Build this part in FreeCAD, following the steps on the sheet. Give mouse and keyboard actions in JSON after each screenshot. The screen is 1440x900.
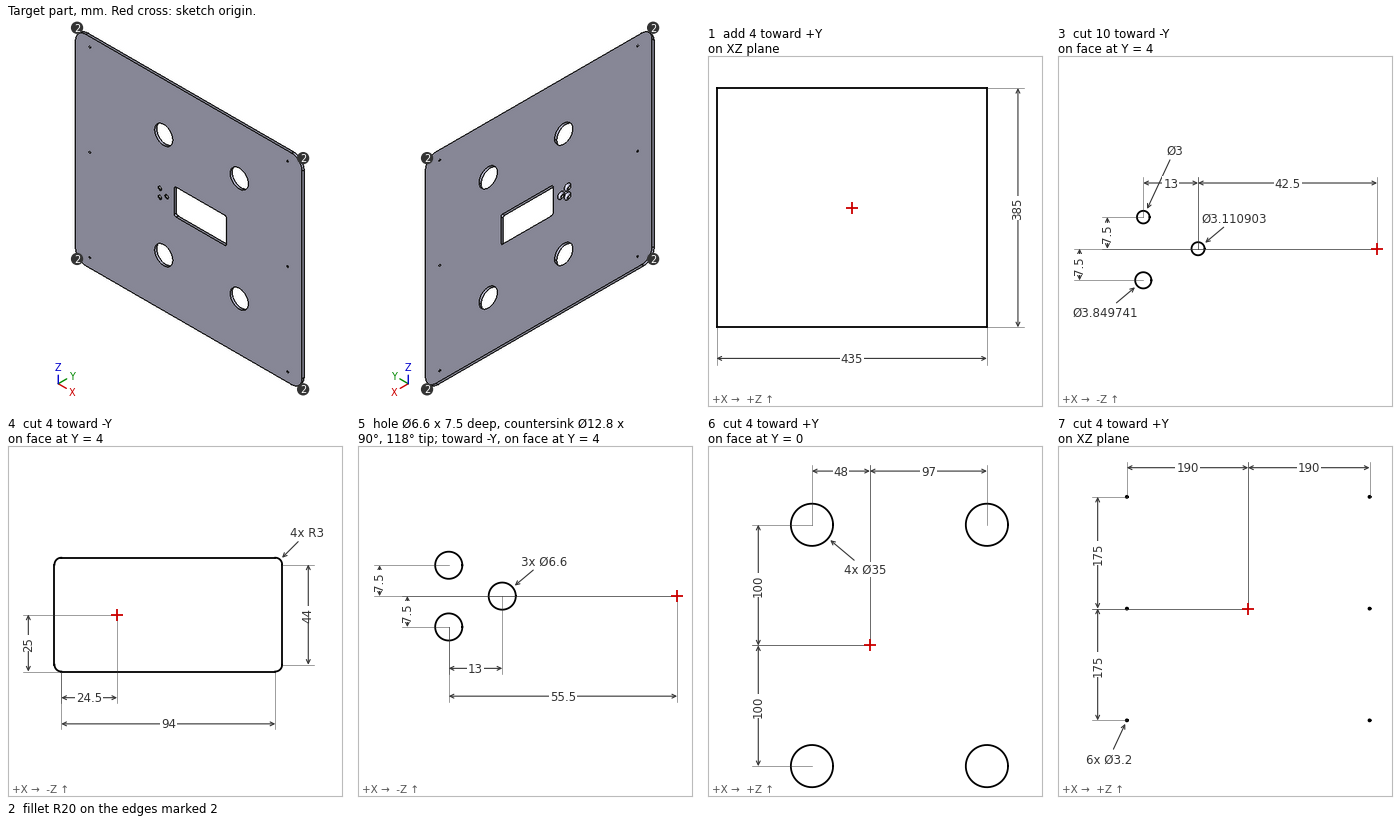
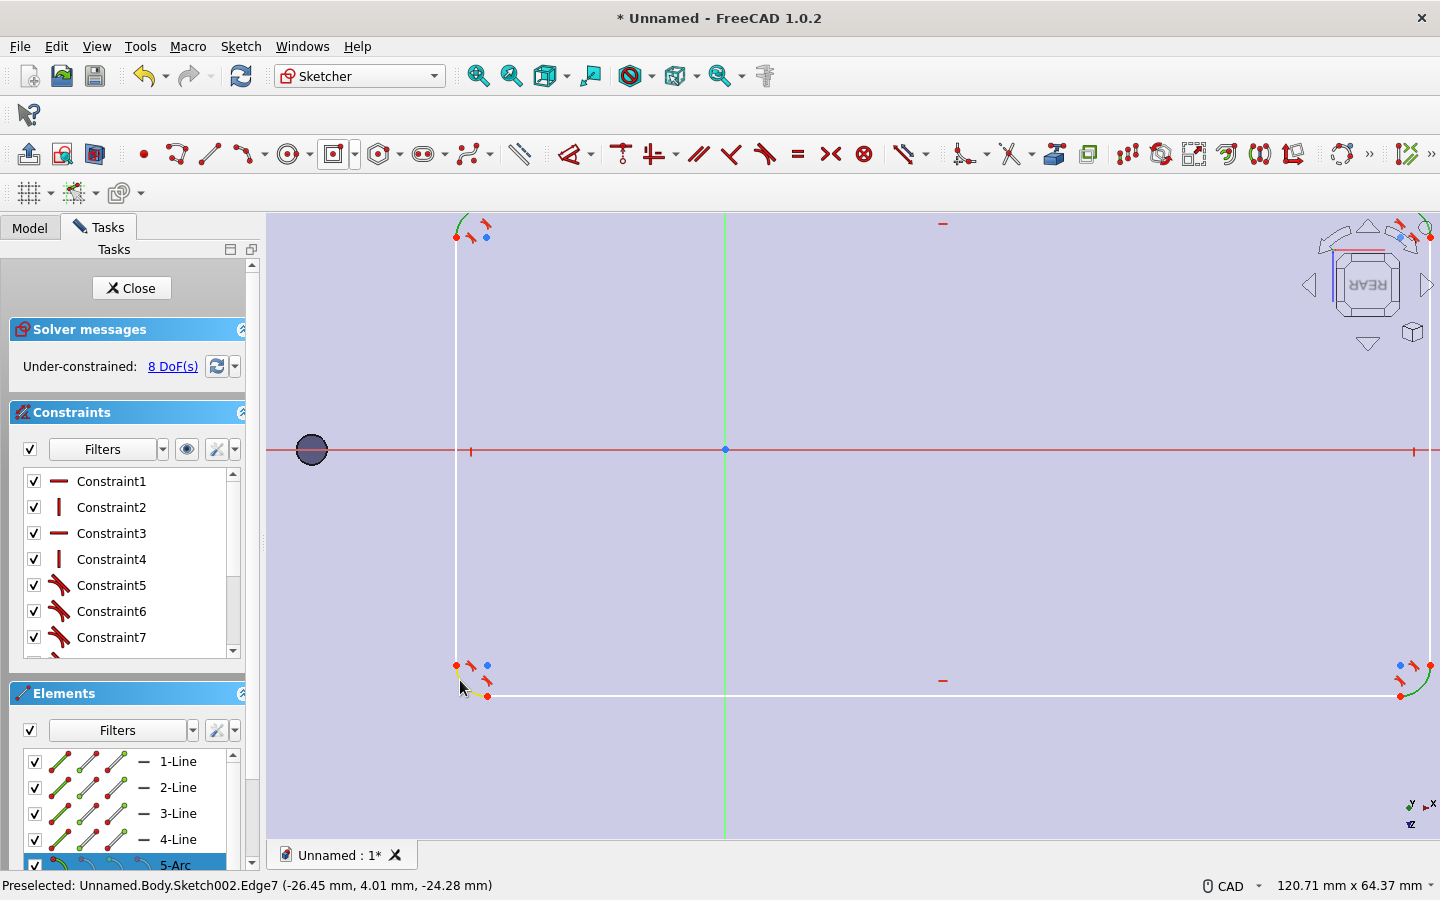
{"action": "left_click", "coordinate": [460, 679]}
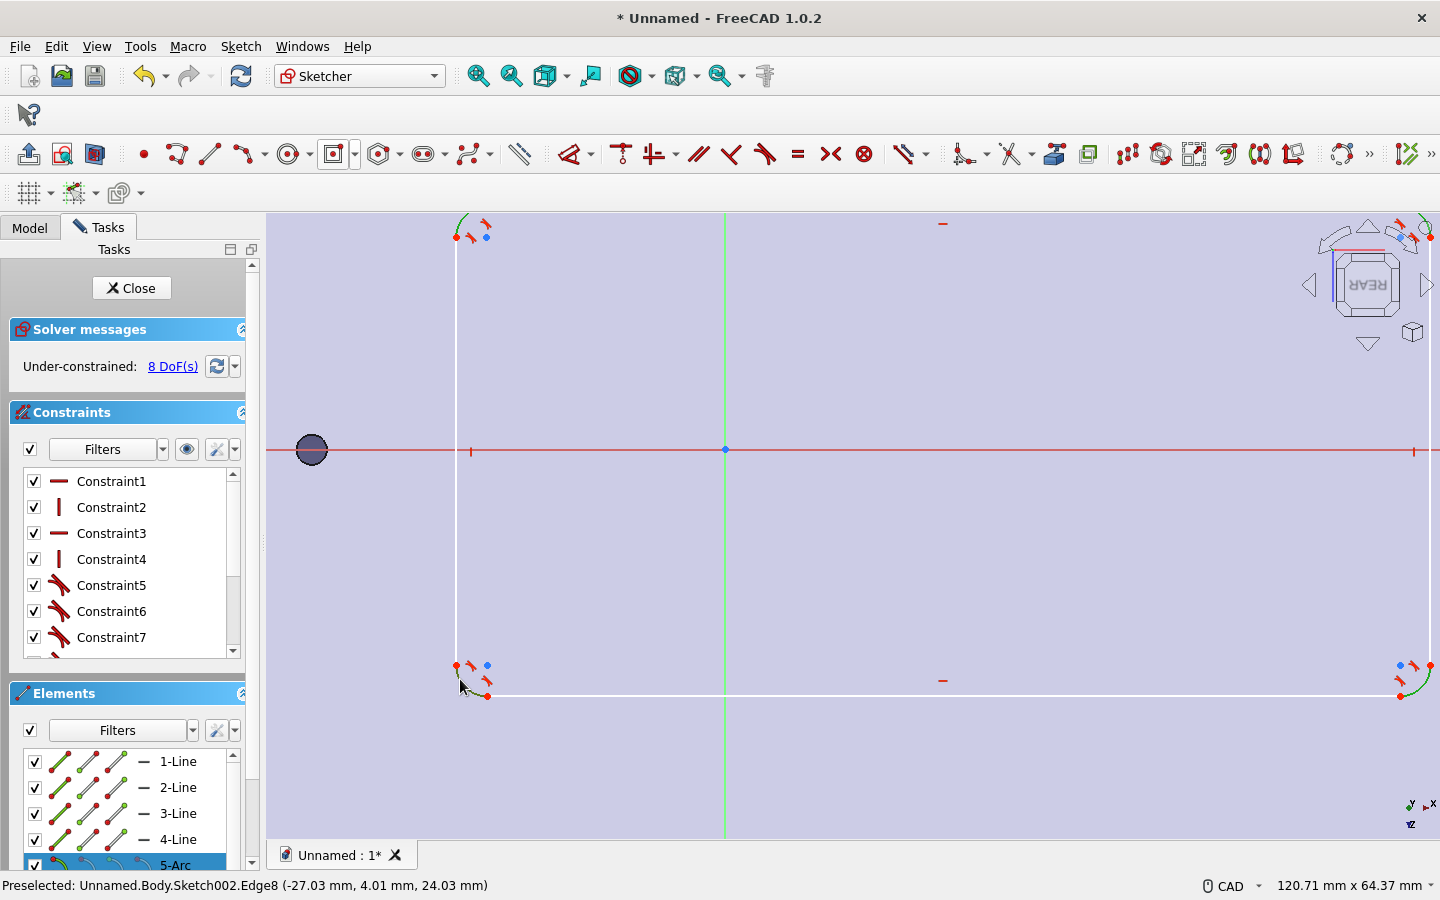
{"action": "left_click", "coordinate": [798, 154]}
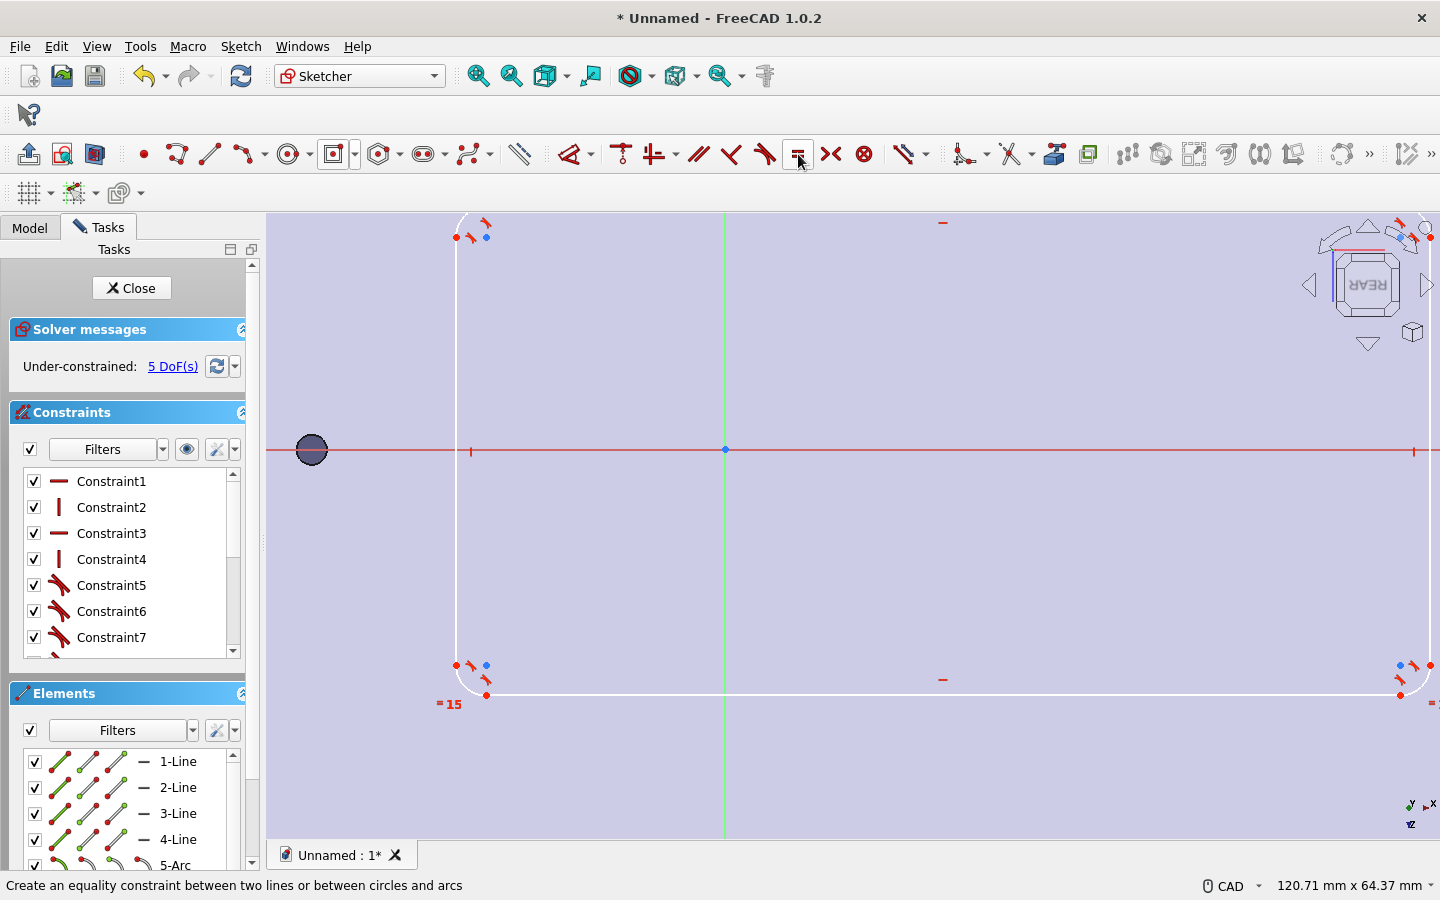
{"action": "left_click", "coordinate": [568, 154]}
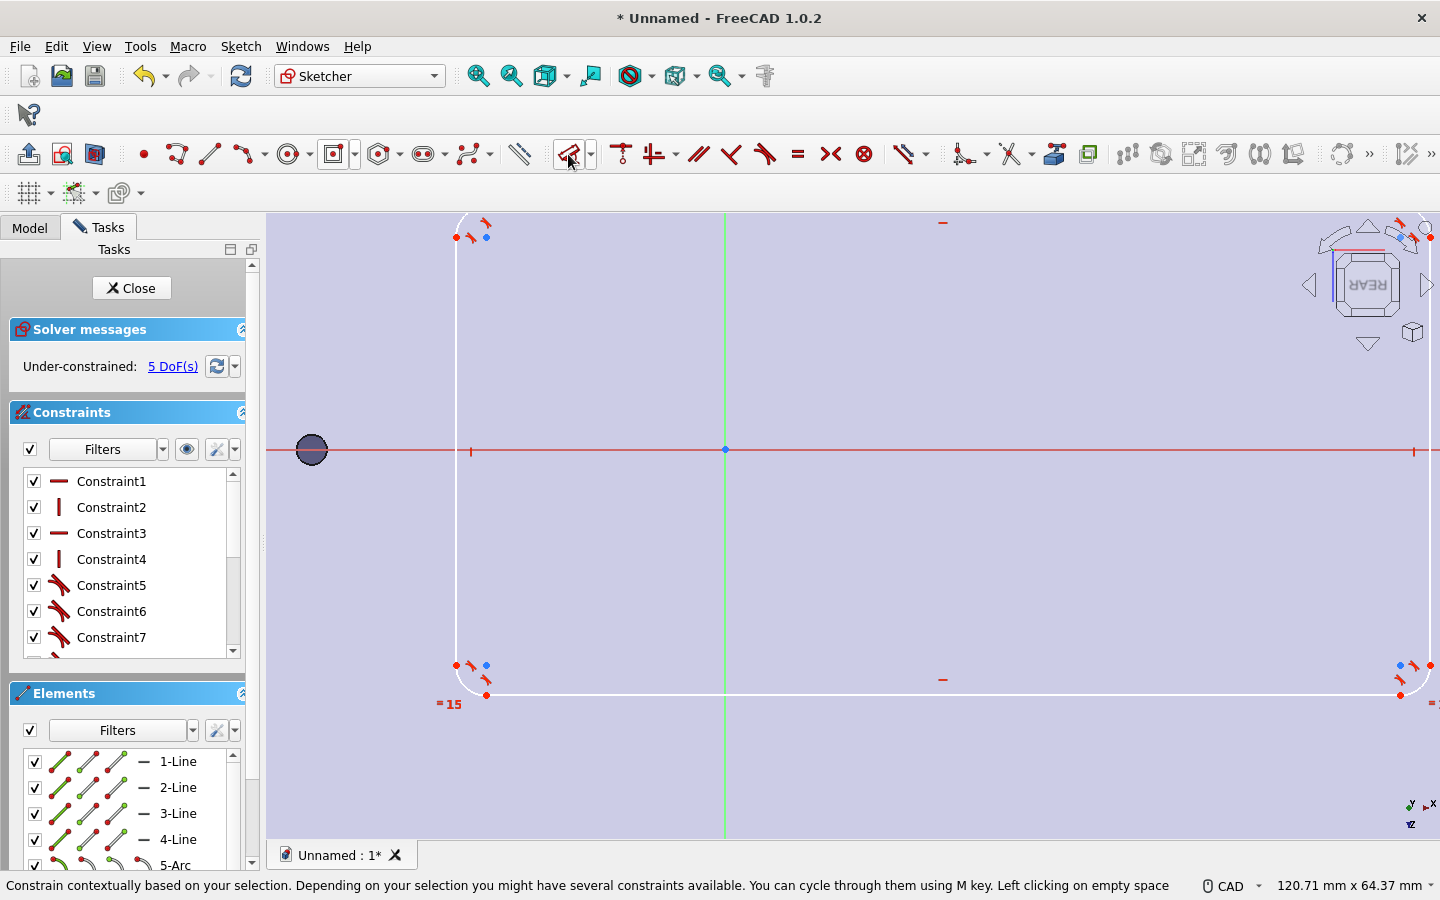
{"action": "scroll", "coordinate": [460, 681], "scroll_direction": "down", "scroll_amount": 2}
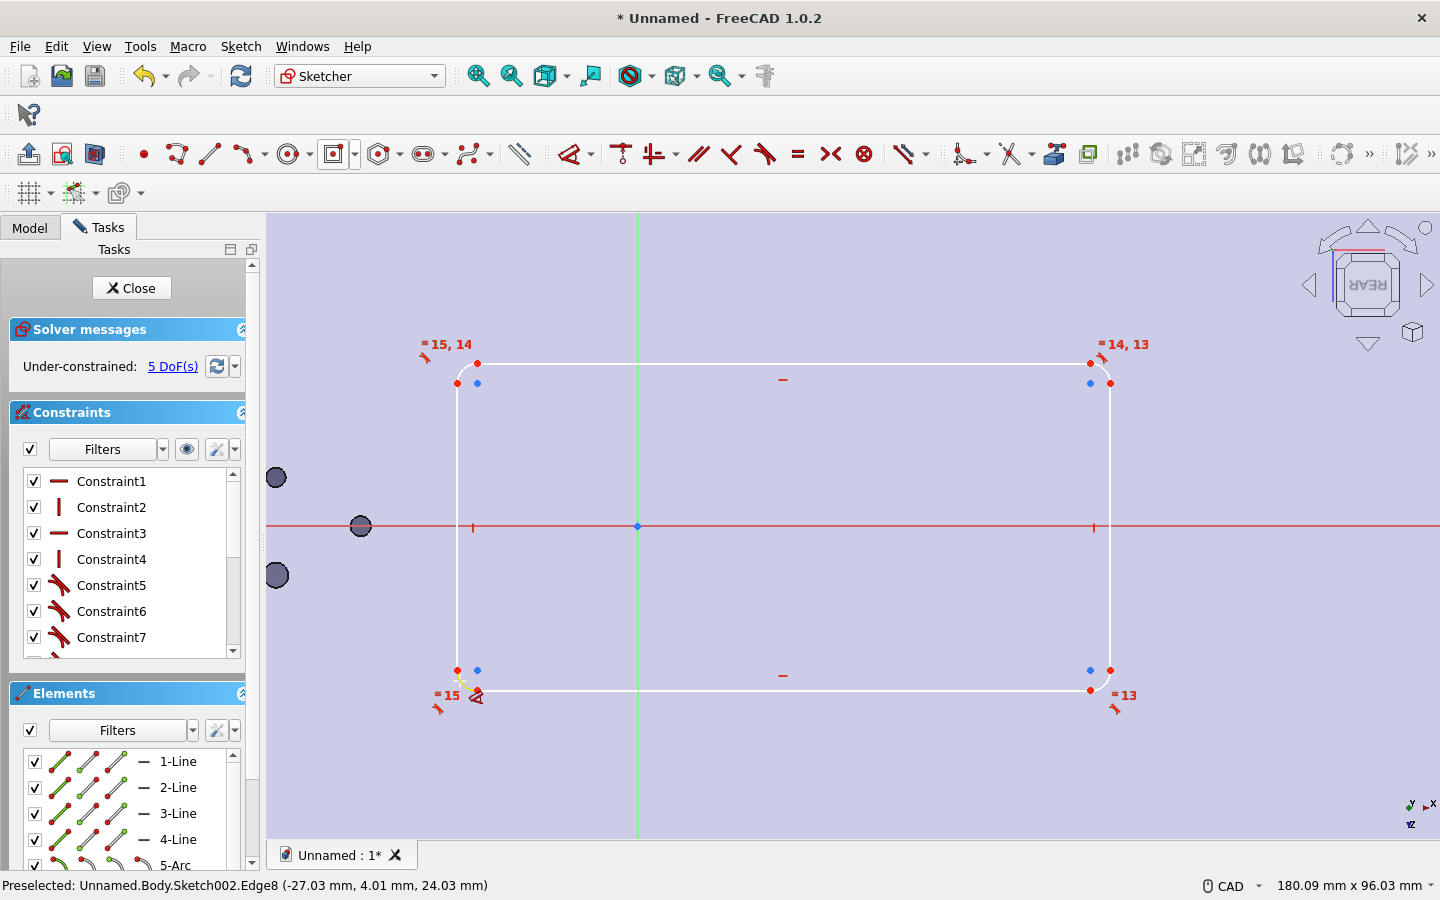
{"action": "scroll", "coordinate": [1099, 689], "scroll_direction": "up", "scroll_amount": 4}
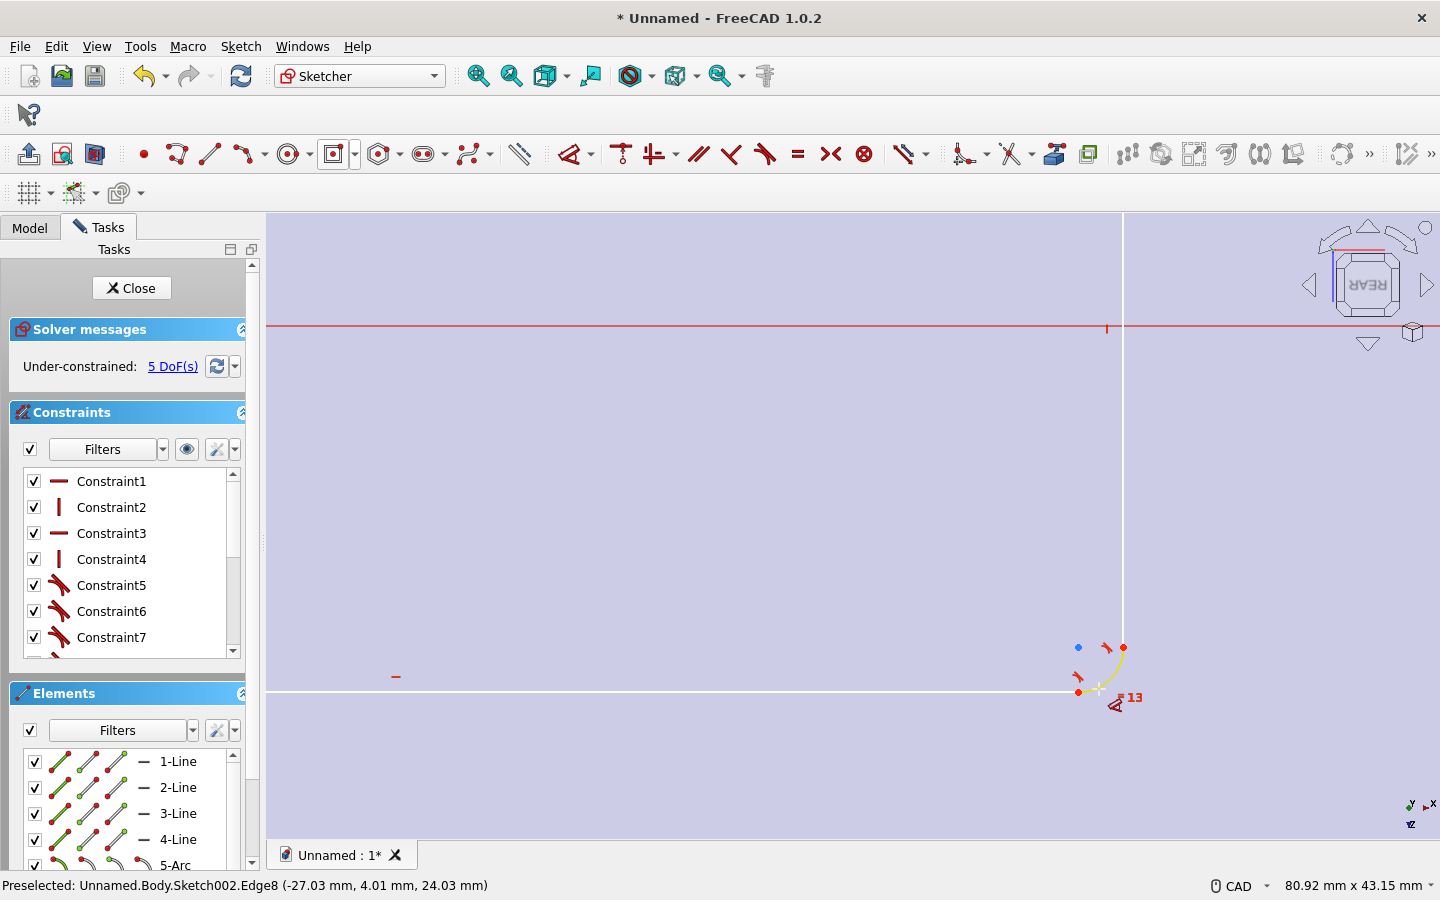
{"action": "left_click", "coordinate": [1099, 688]}
{"action": "left_click", "coordinate": [1113, 717]}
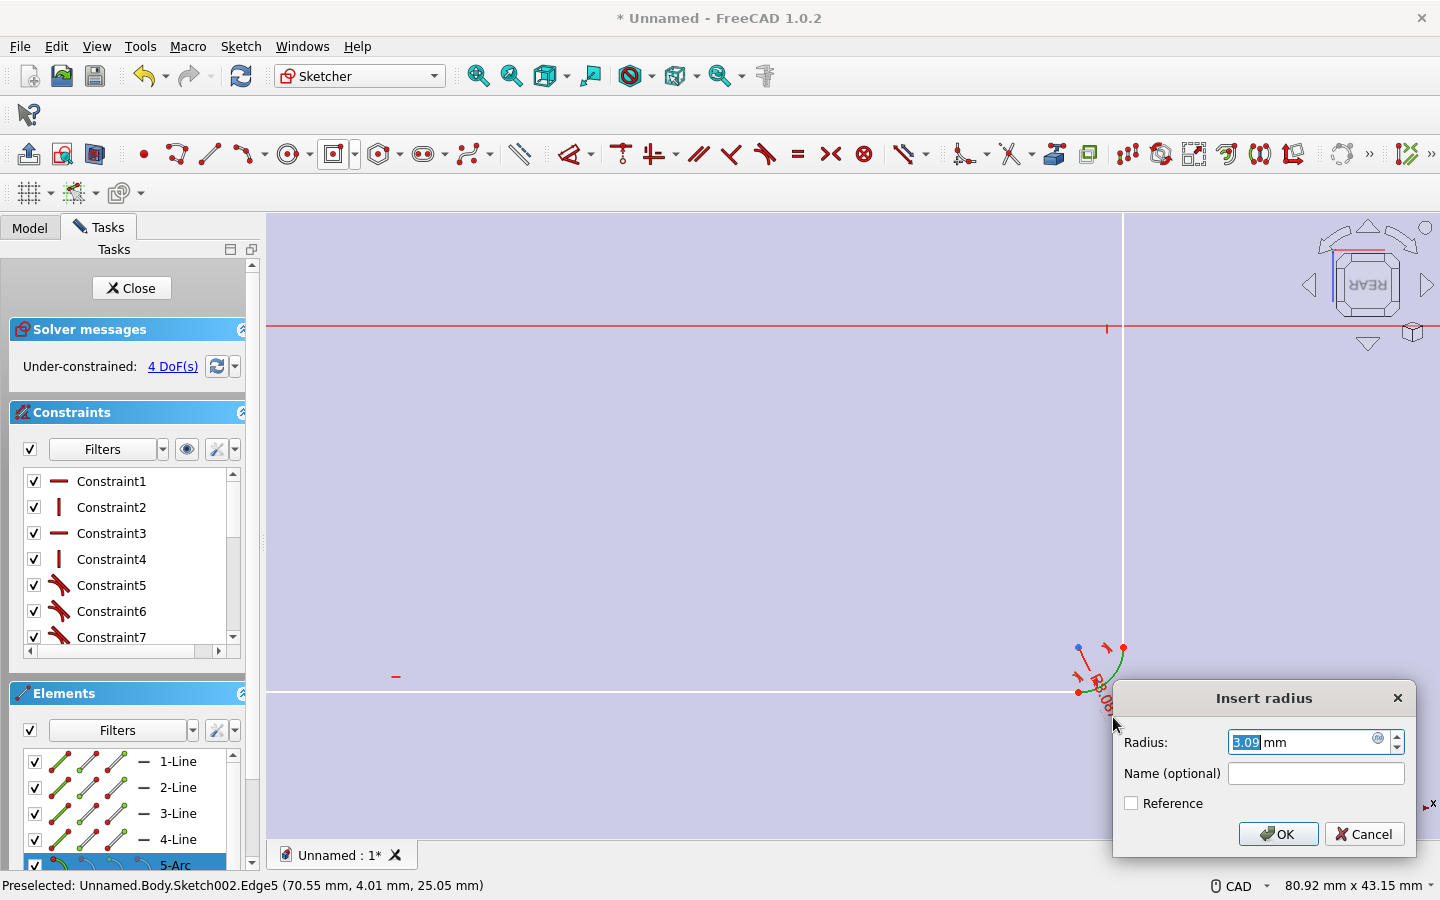
{"action": "type", "text": "3"}
{"action": "key", "text": "Return"}